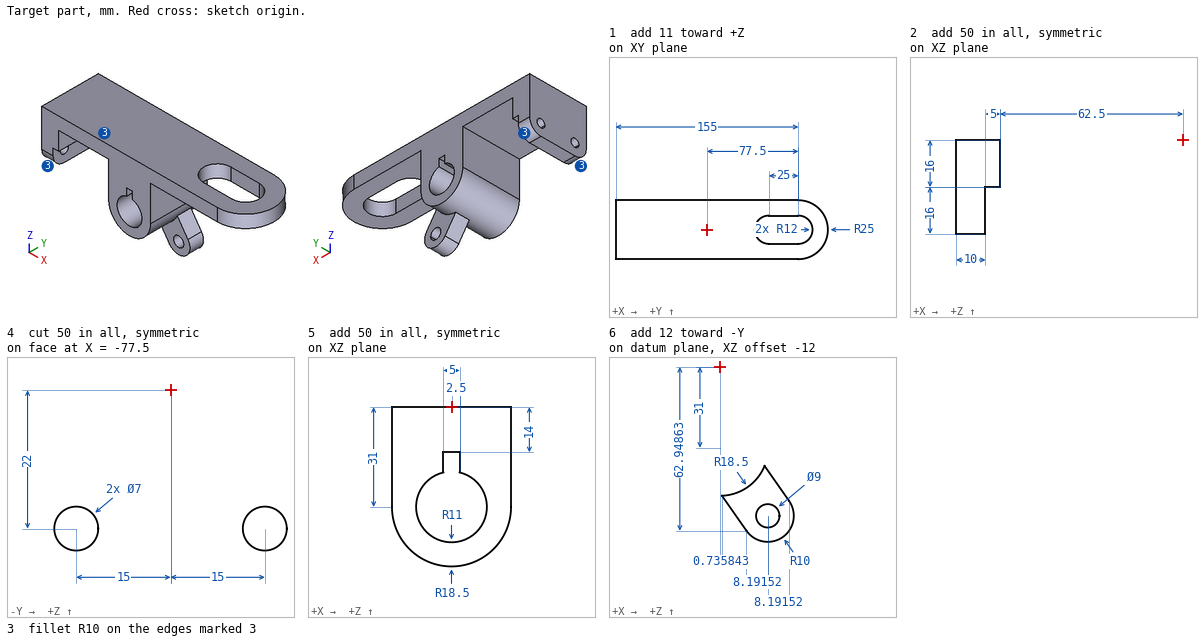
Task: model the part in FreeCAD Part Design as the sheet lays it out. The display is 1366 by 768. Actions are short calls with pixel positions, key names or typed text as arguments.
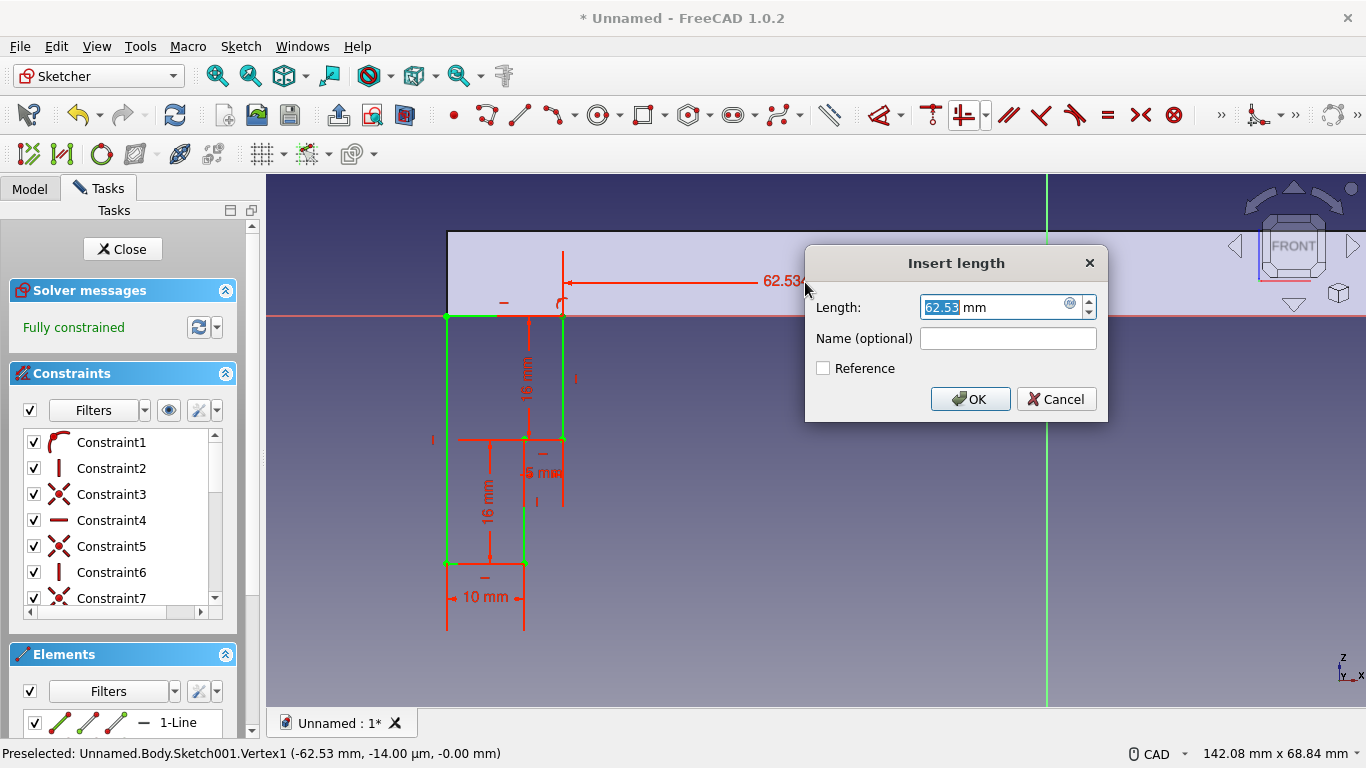
text(62.5)
key(Return)
key(Escape)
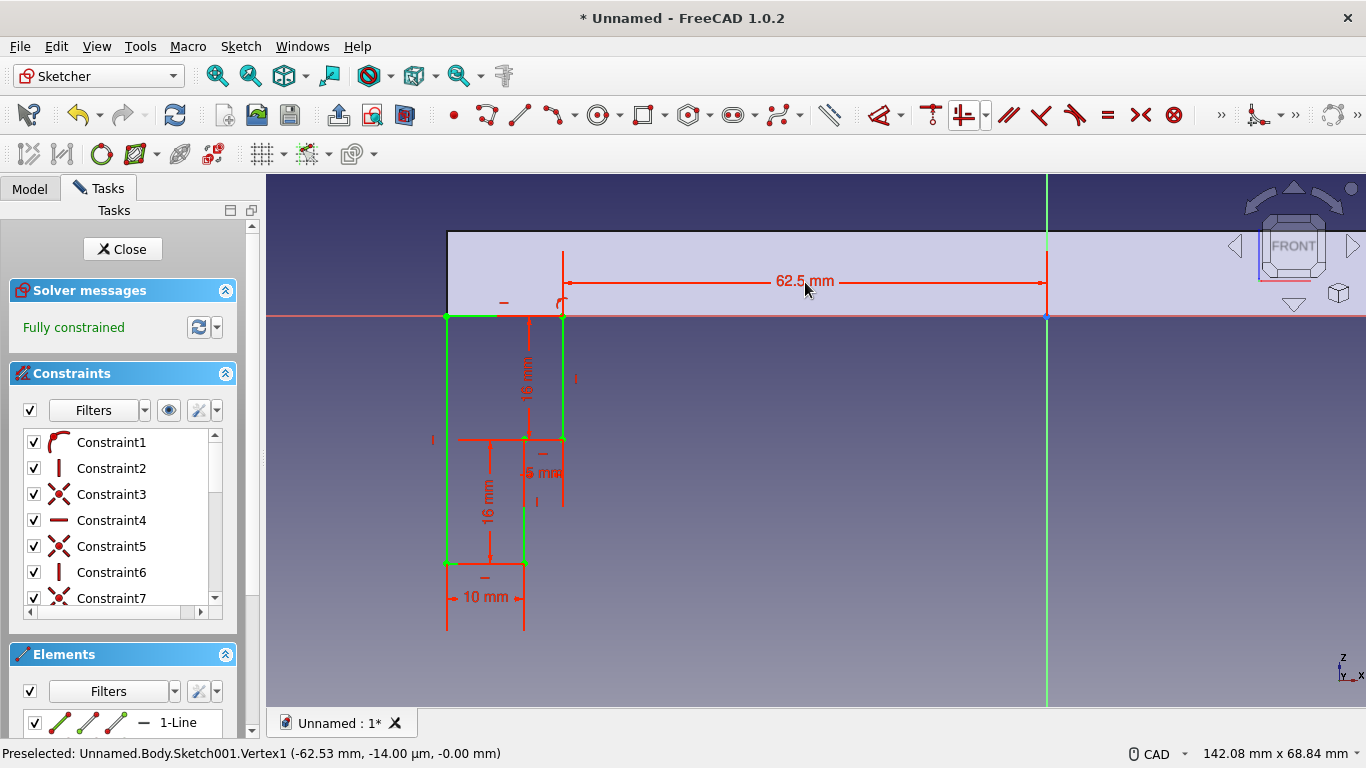
click(123, 249)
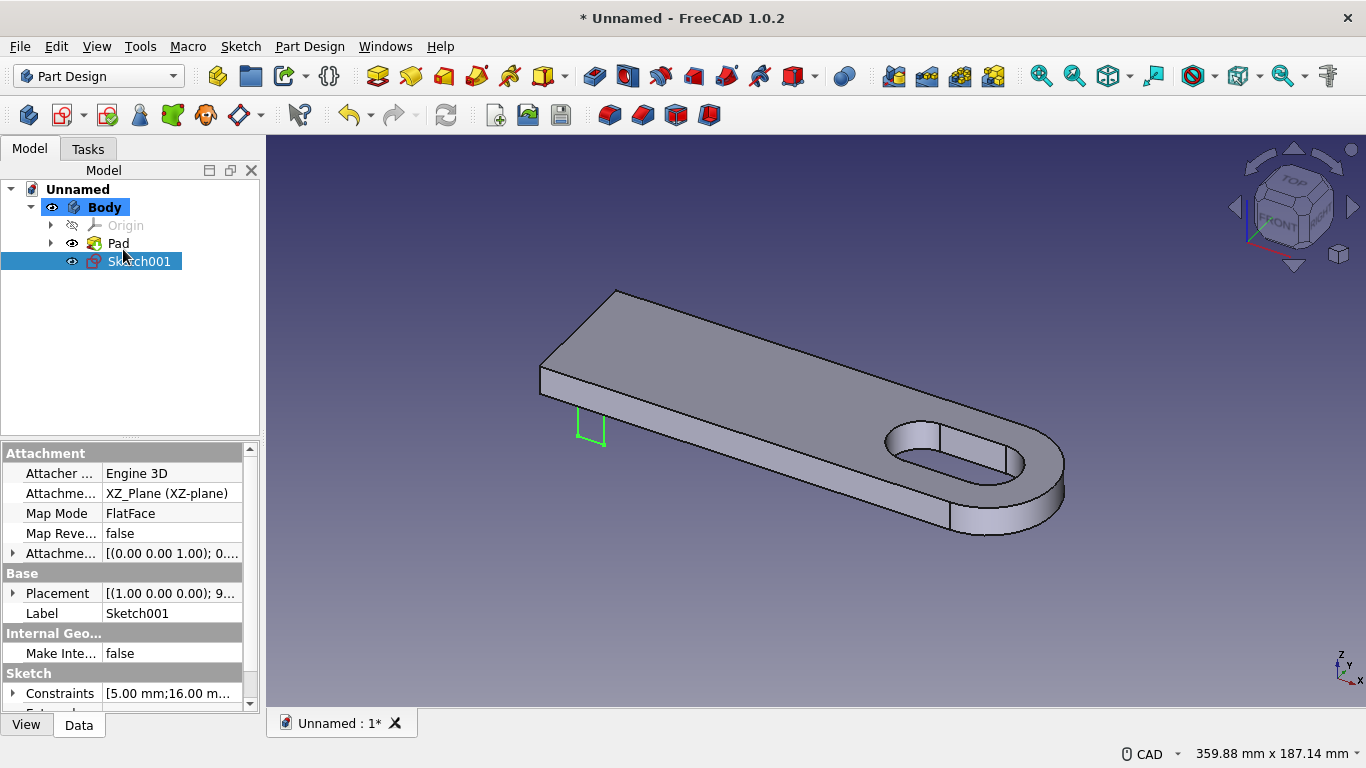
click(378, 76)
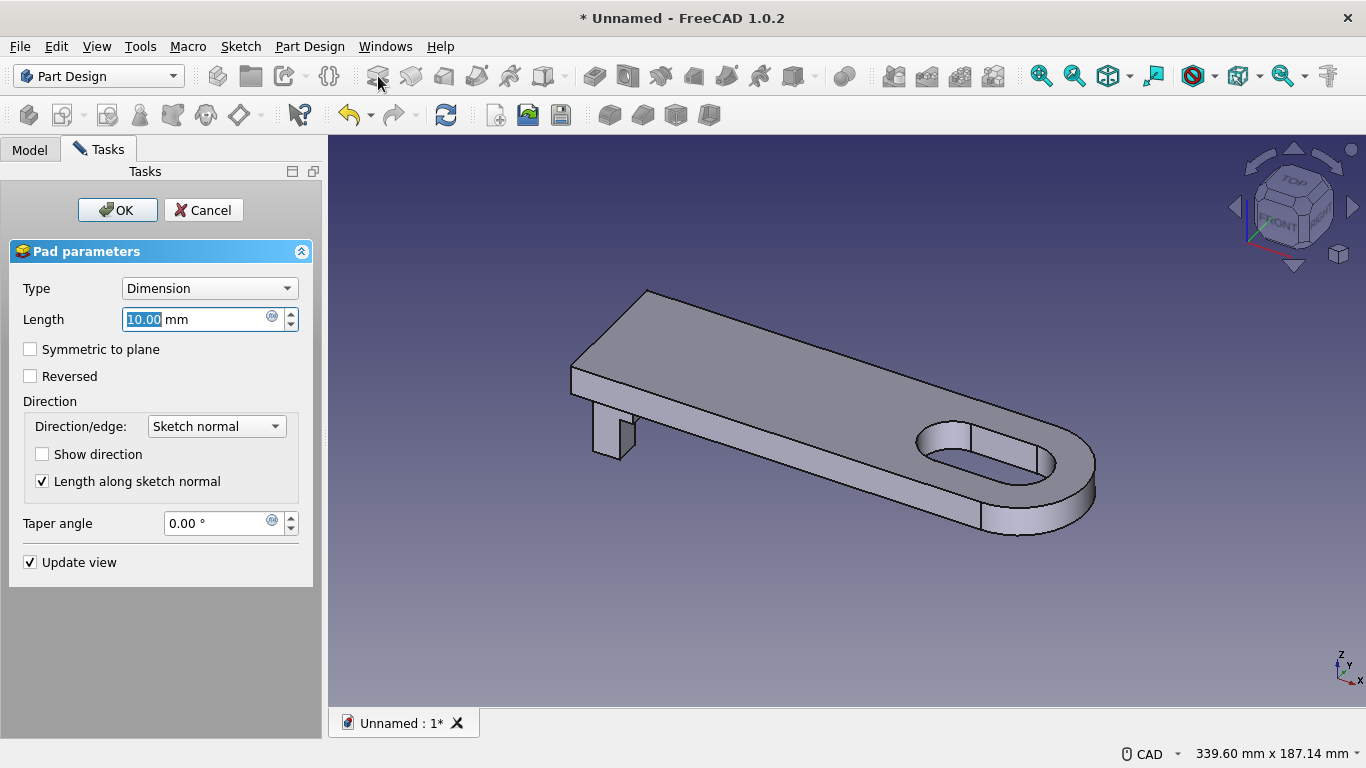
text(50)
key(Tab)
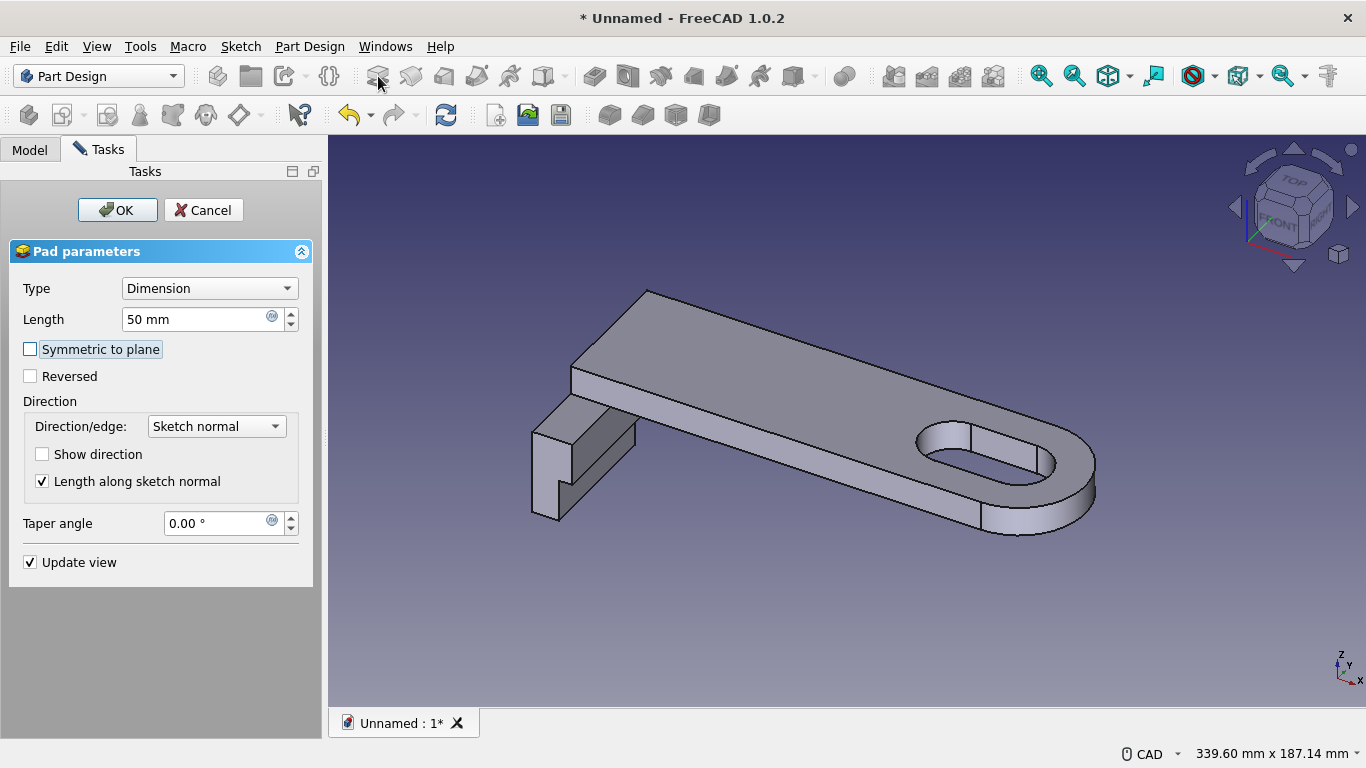
click(31, 349)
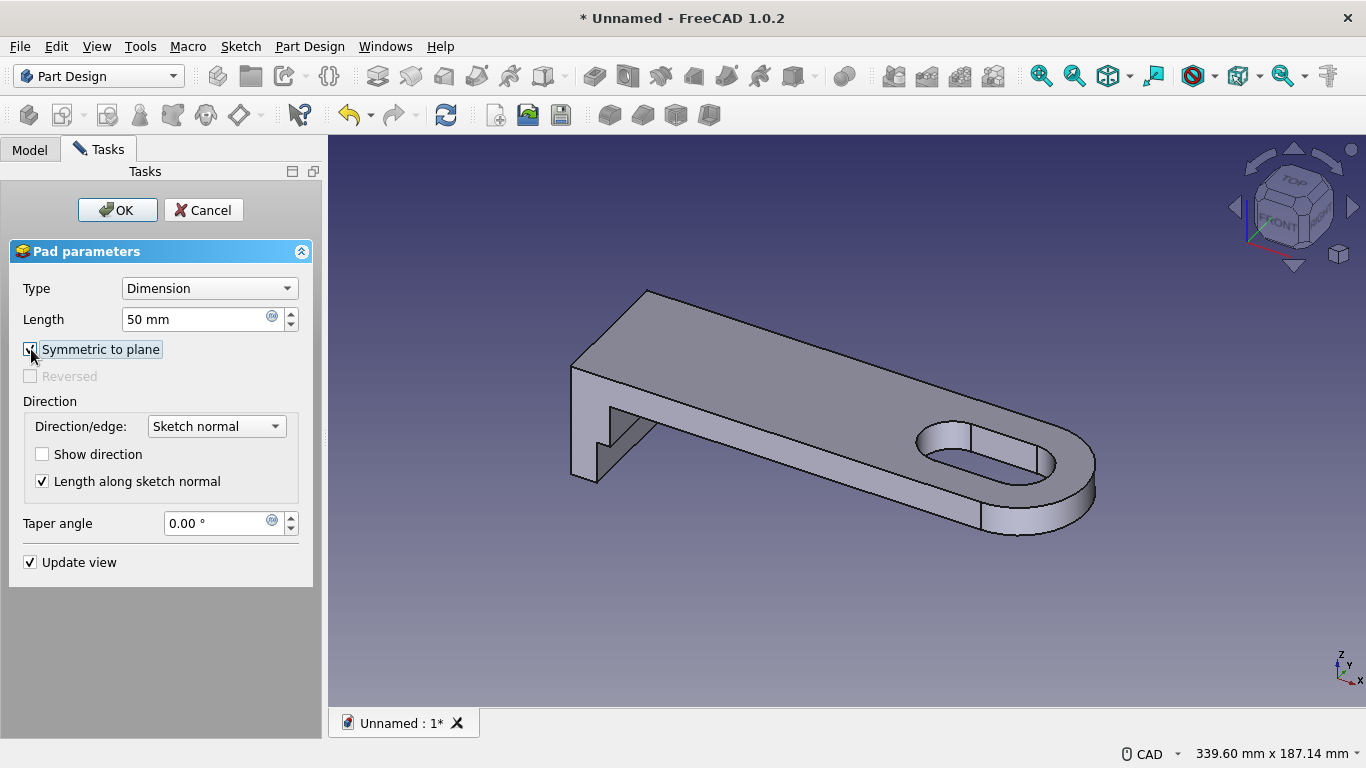
click(118, 210)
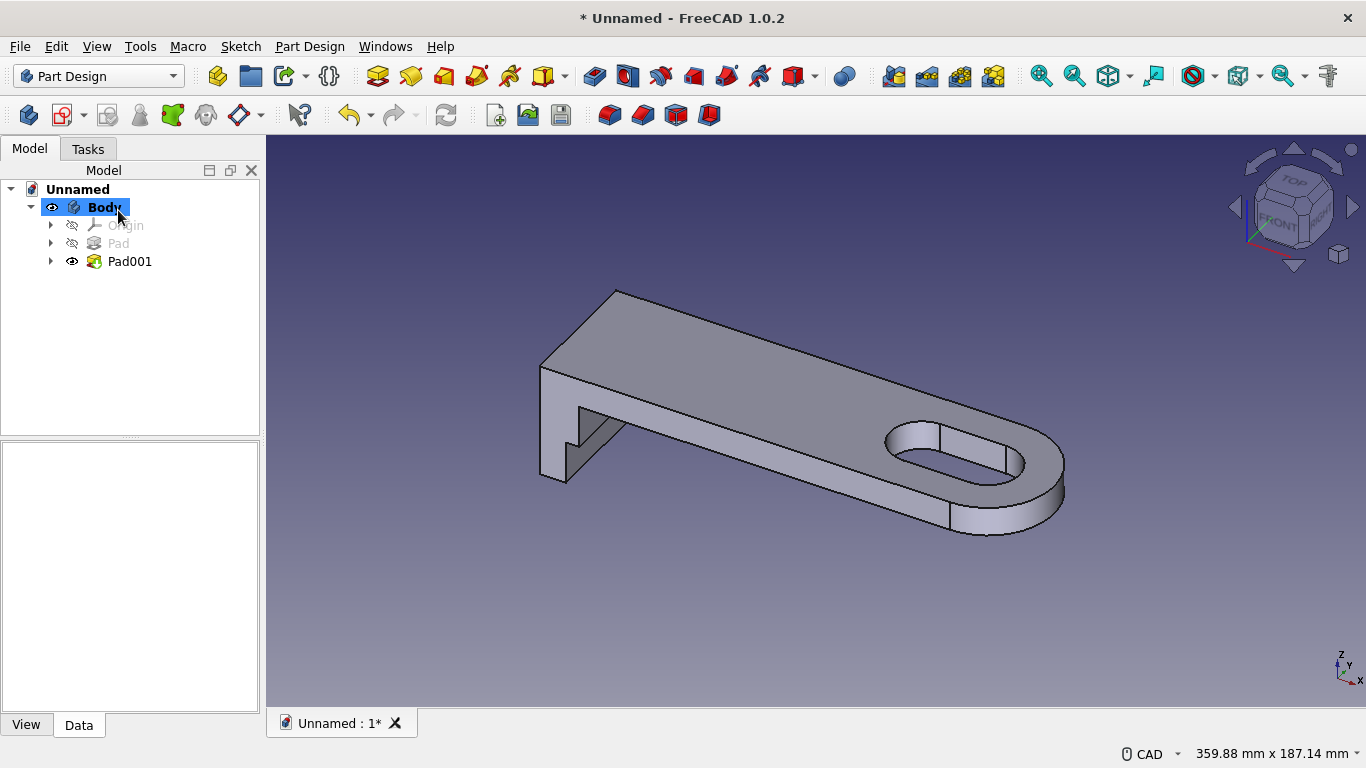
key(0)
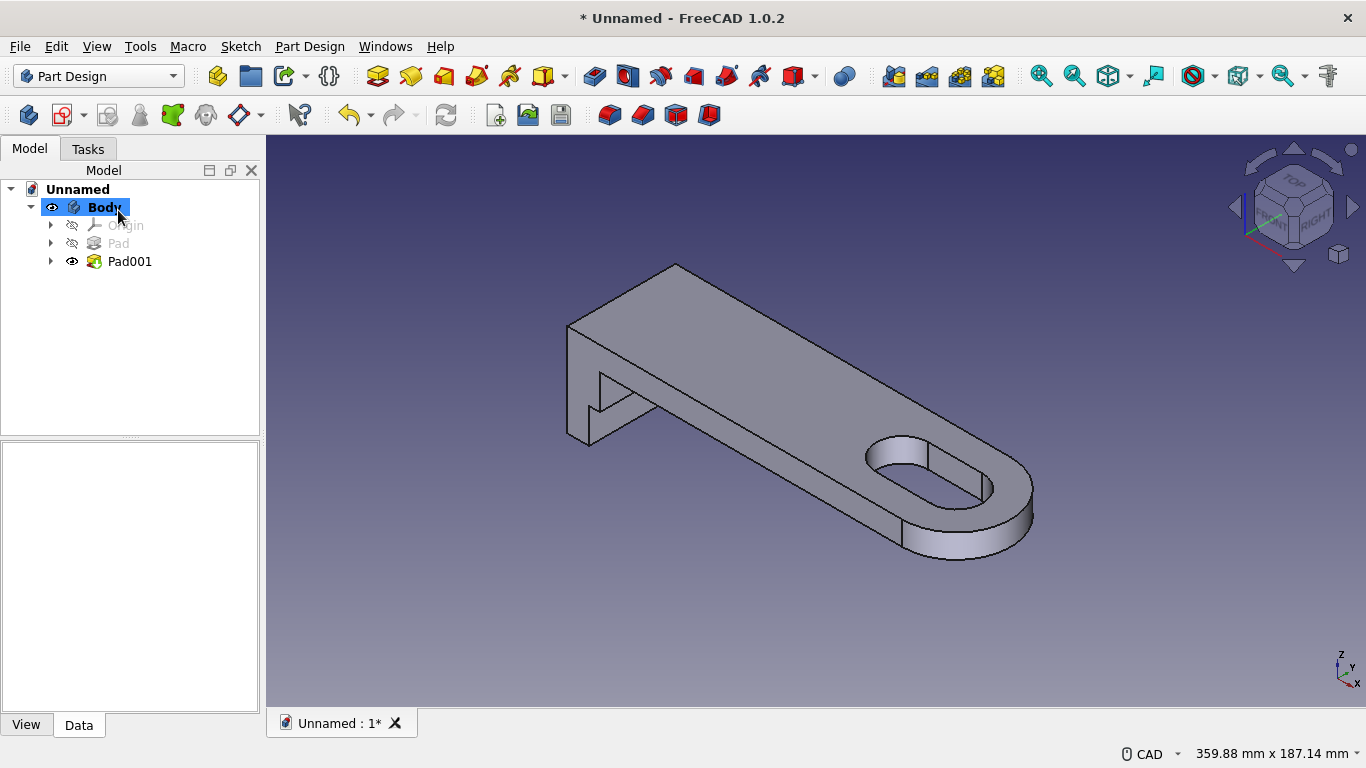
key(2)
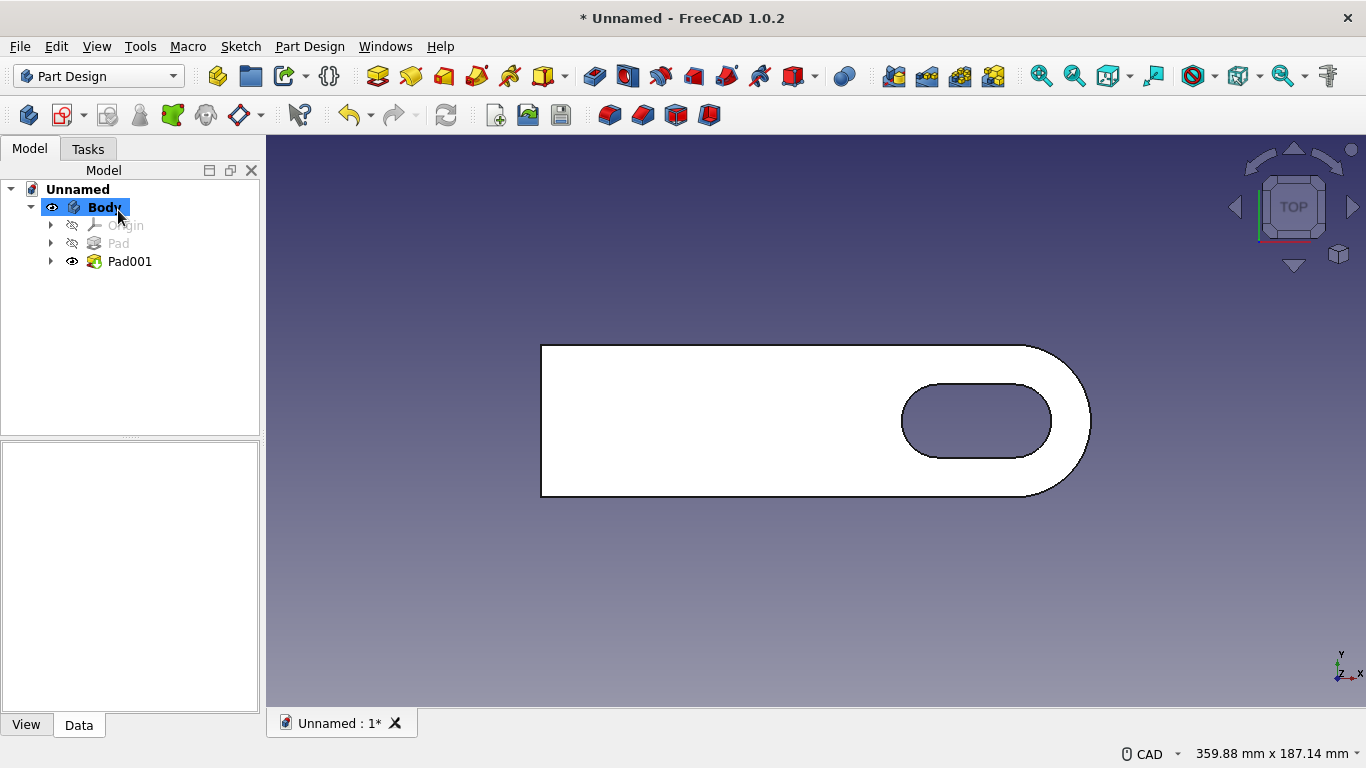
key(1)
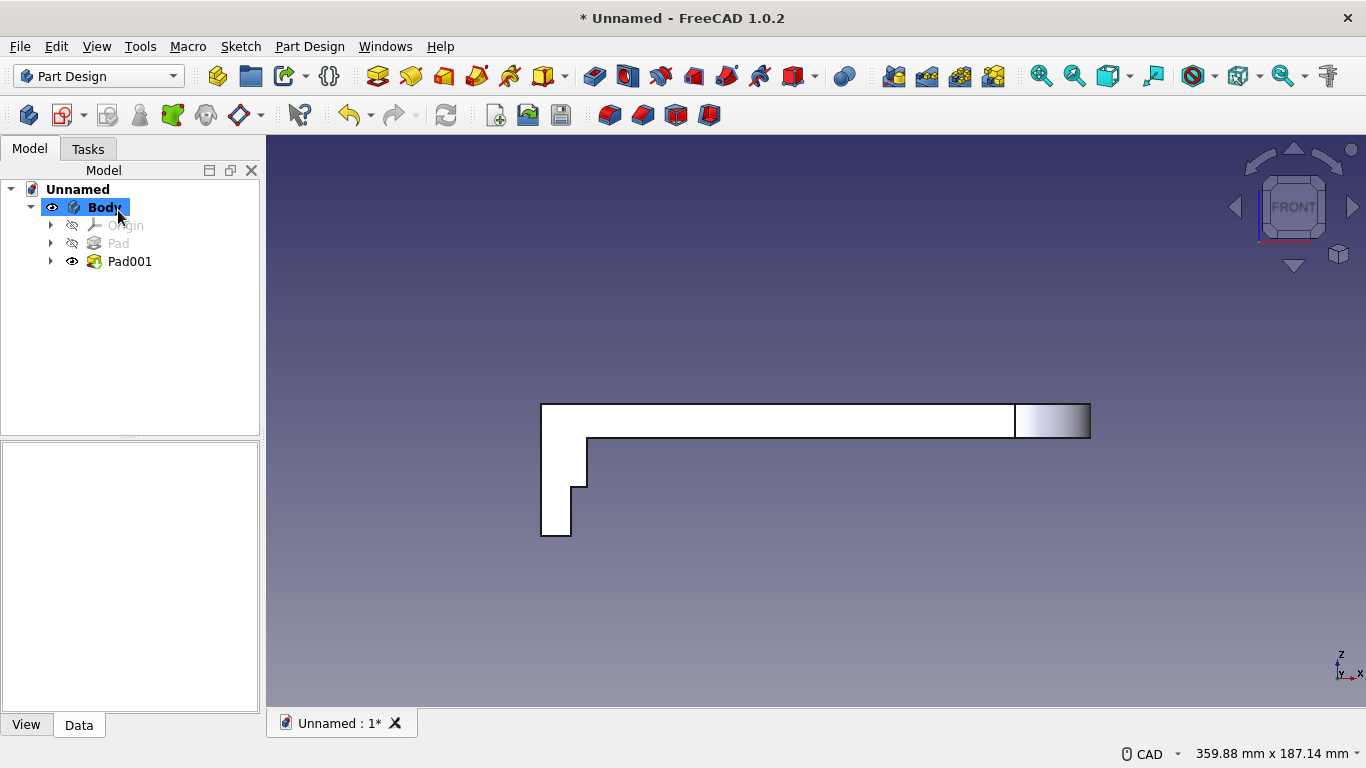
click(556, 535)